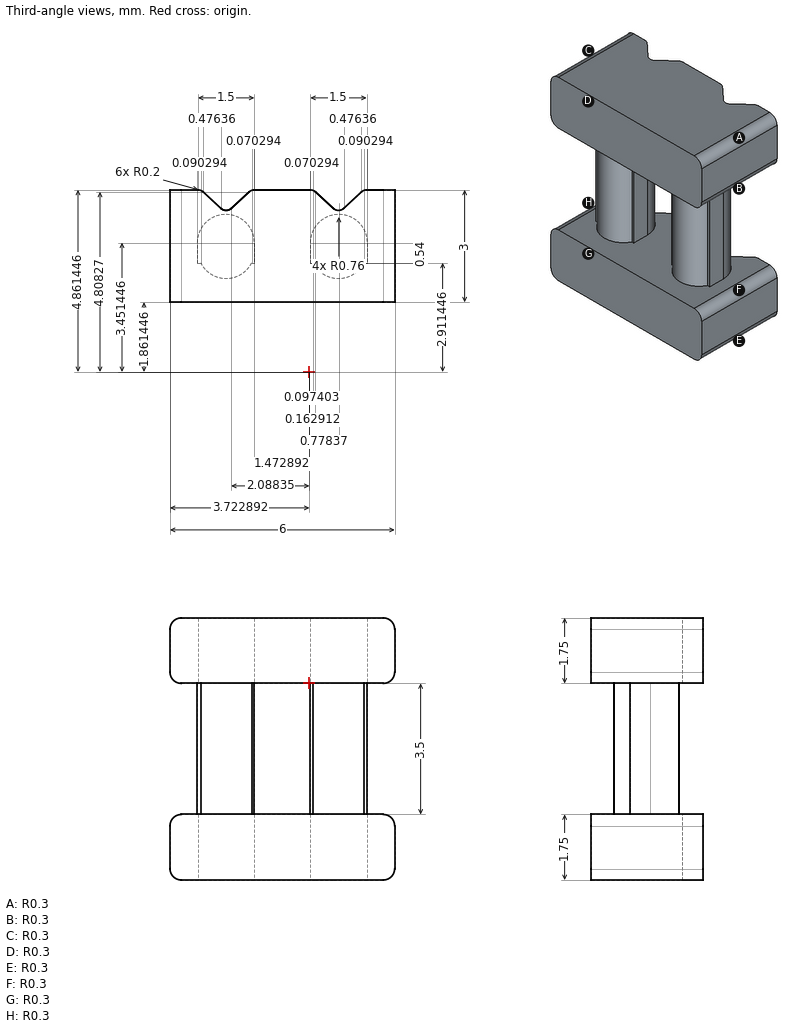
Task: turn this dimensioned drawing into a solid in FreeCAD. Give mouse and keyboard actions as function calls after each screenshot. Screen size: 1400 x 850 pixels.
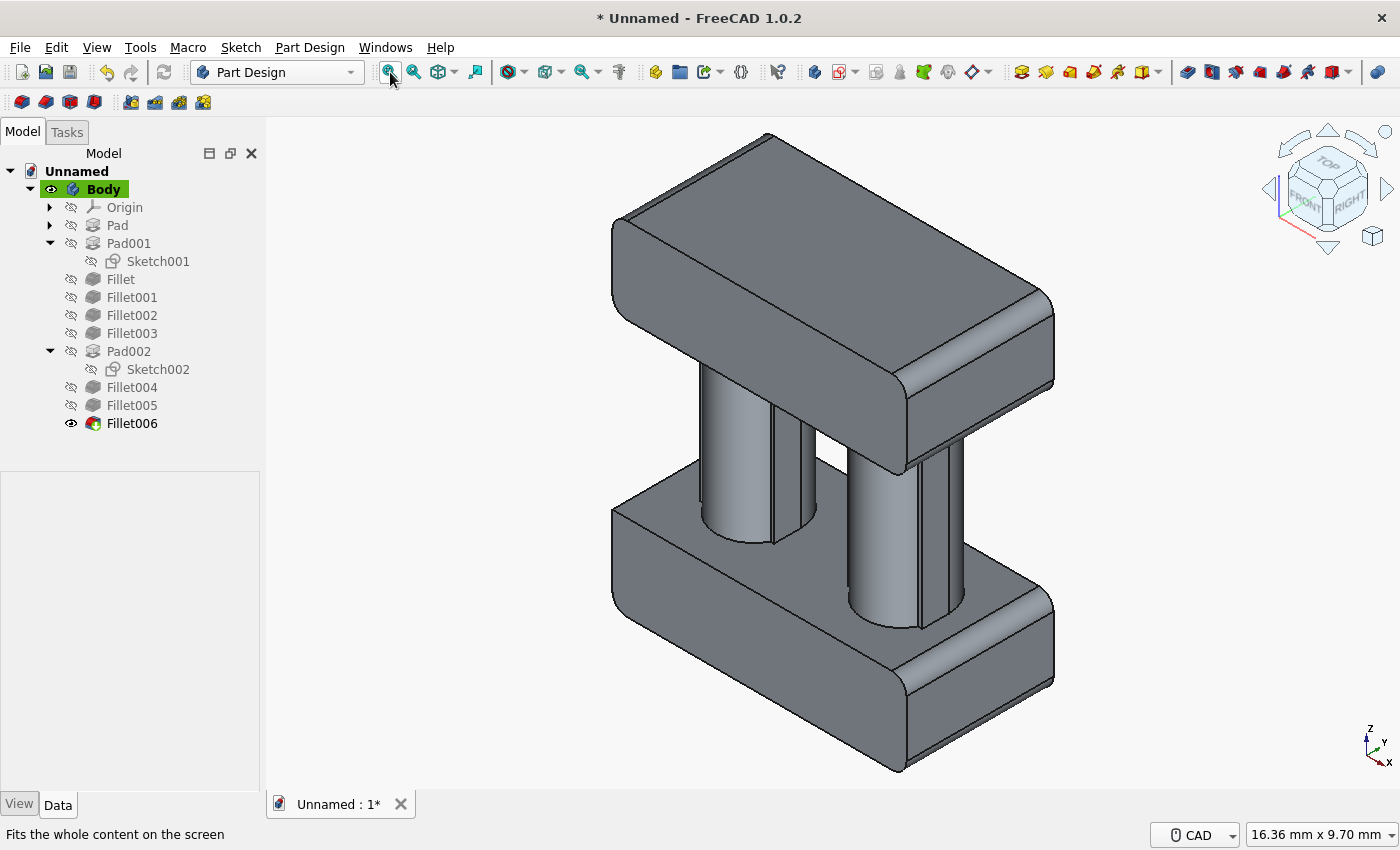
key(2)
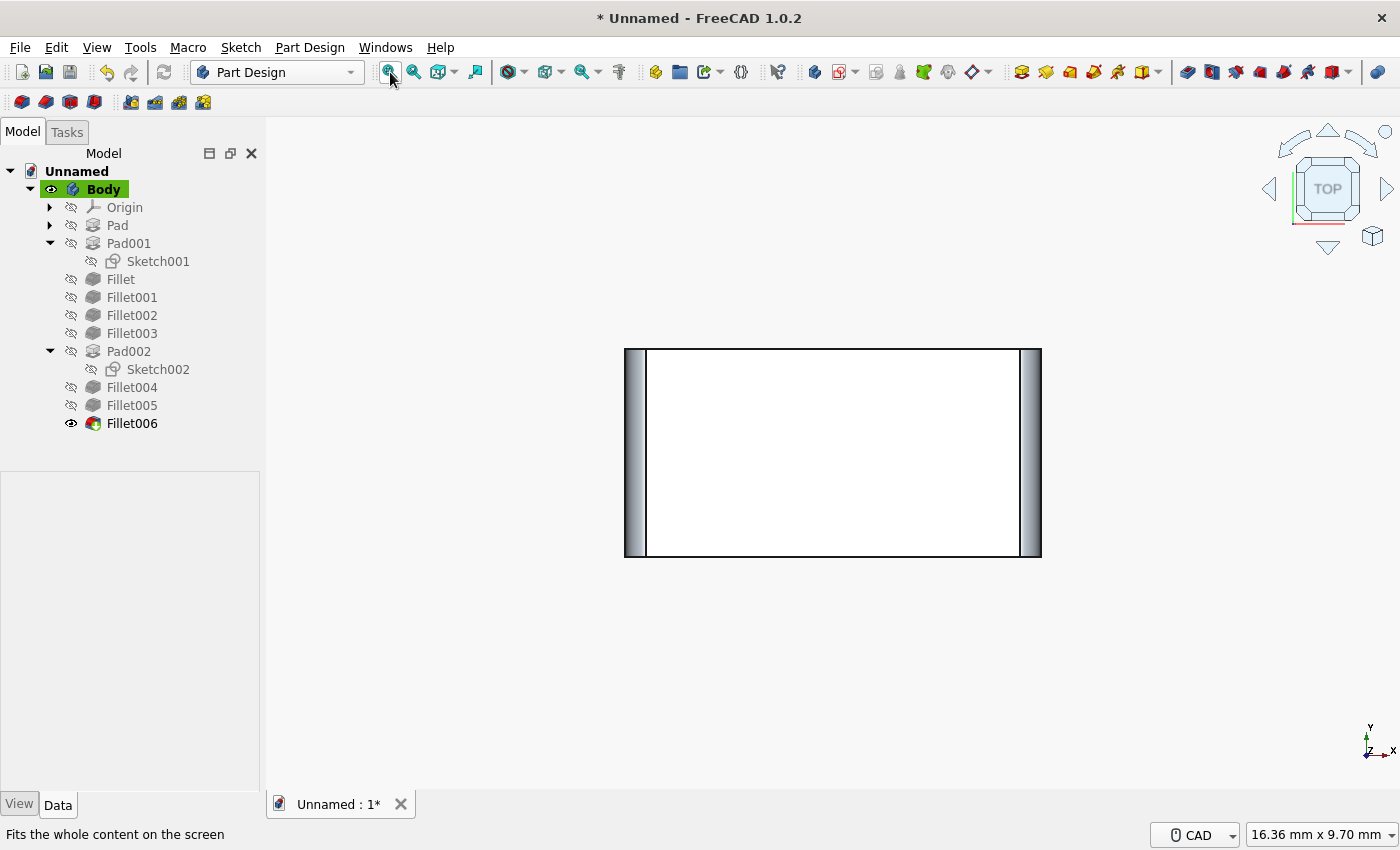
click(390, 72)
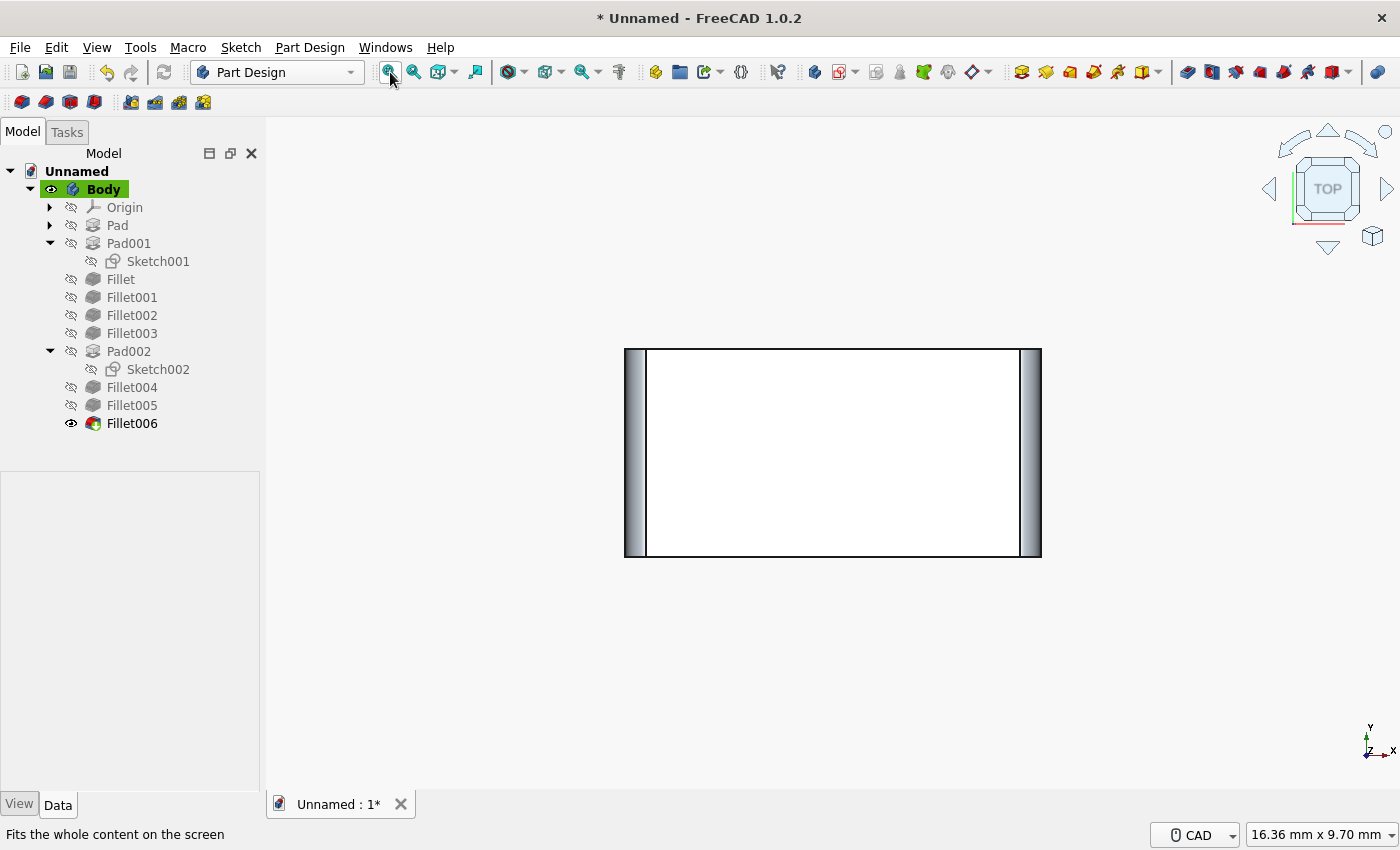
key(1)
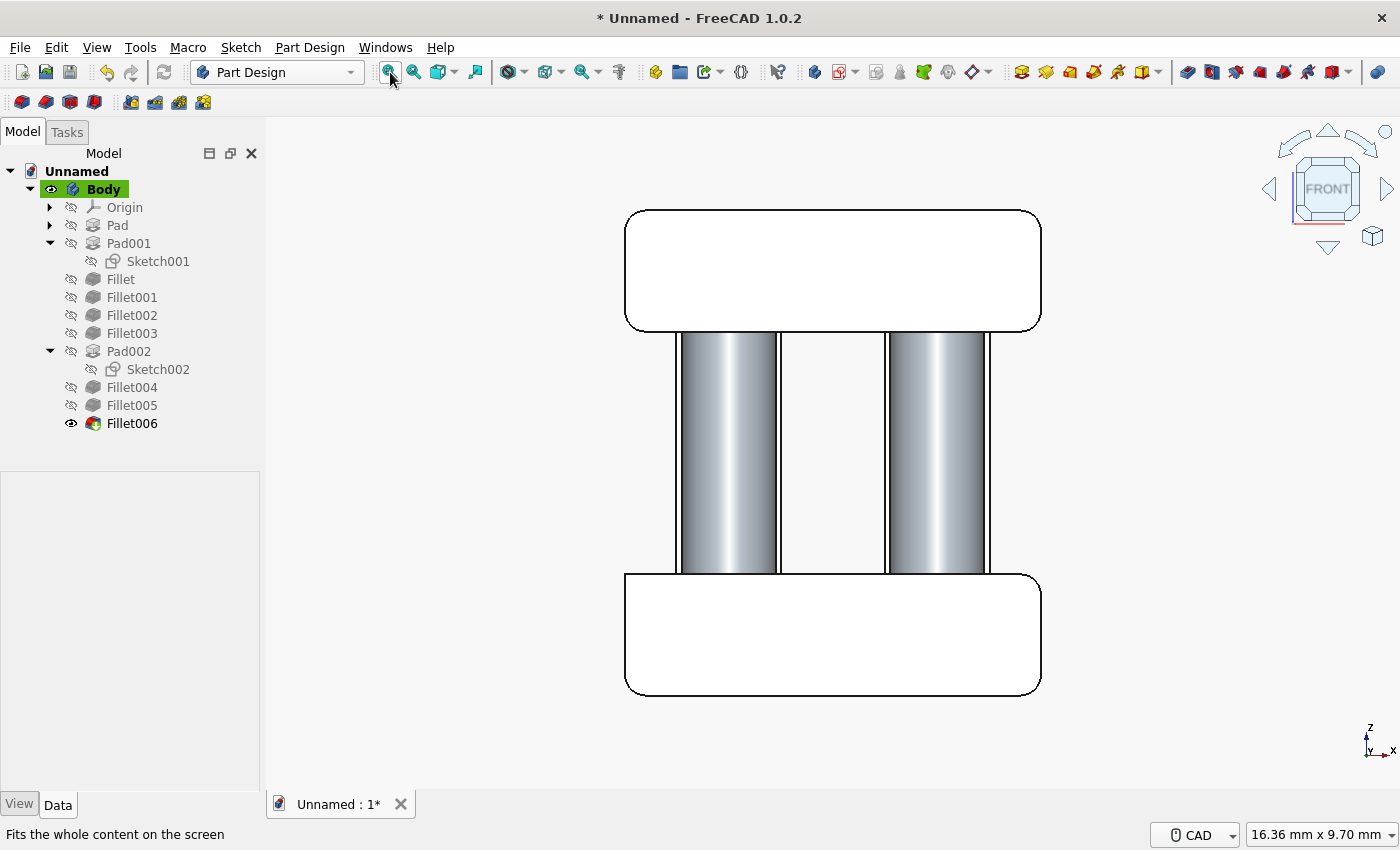
key(3)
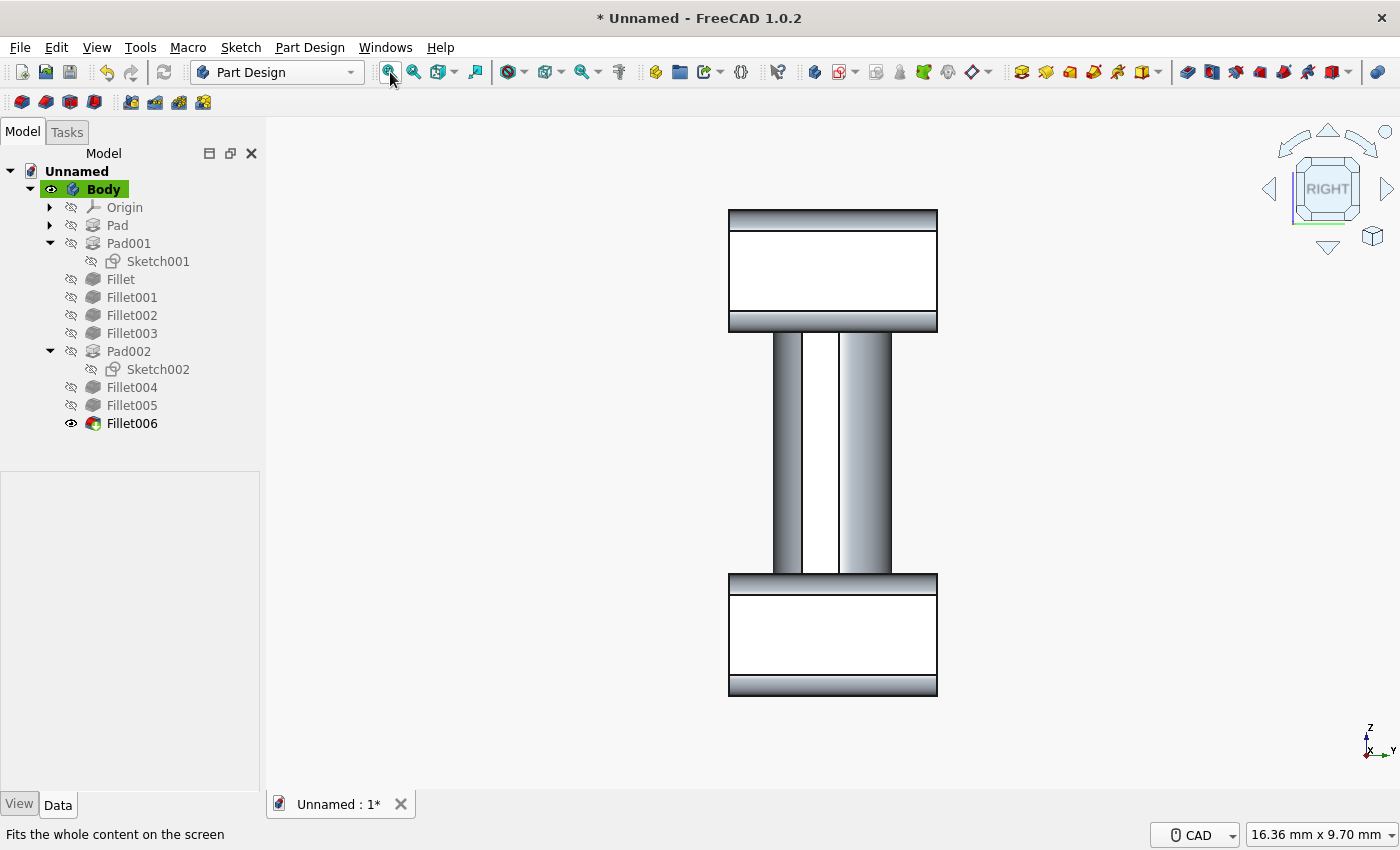
key(5)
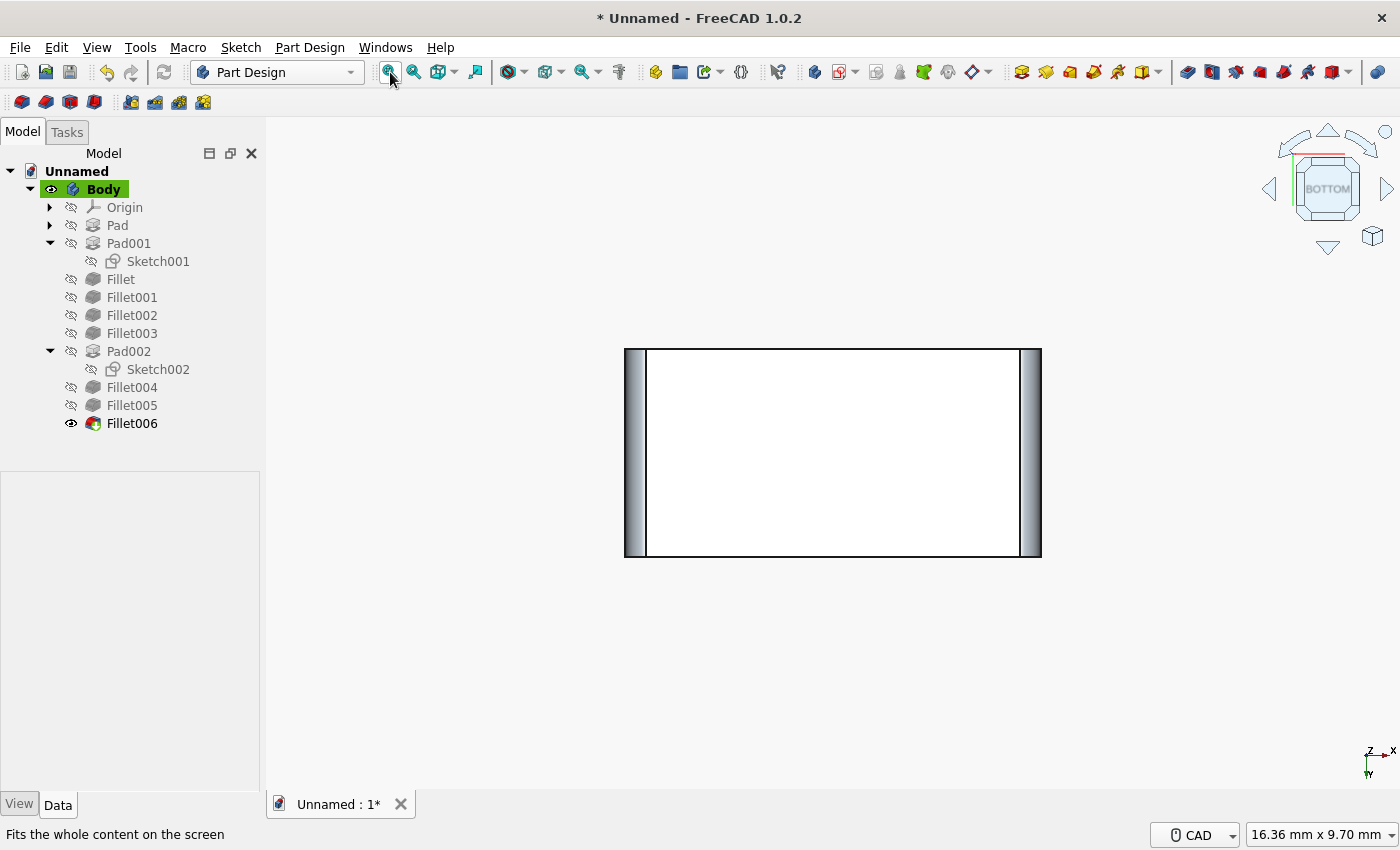
click(390, 72)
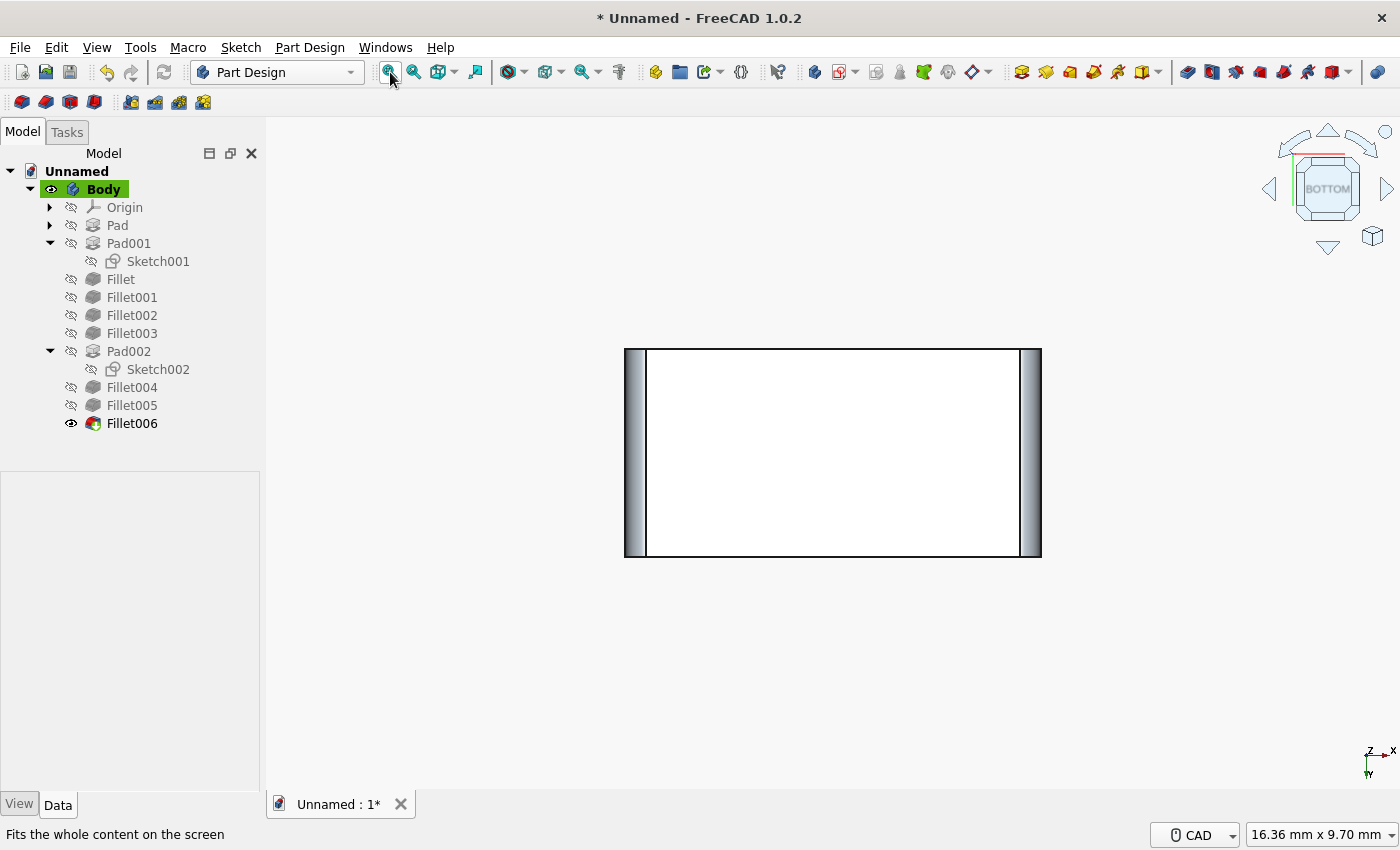
key(4)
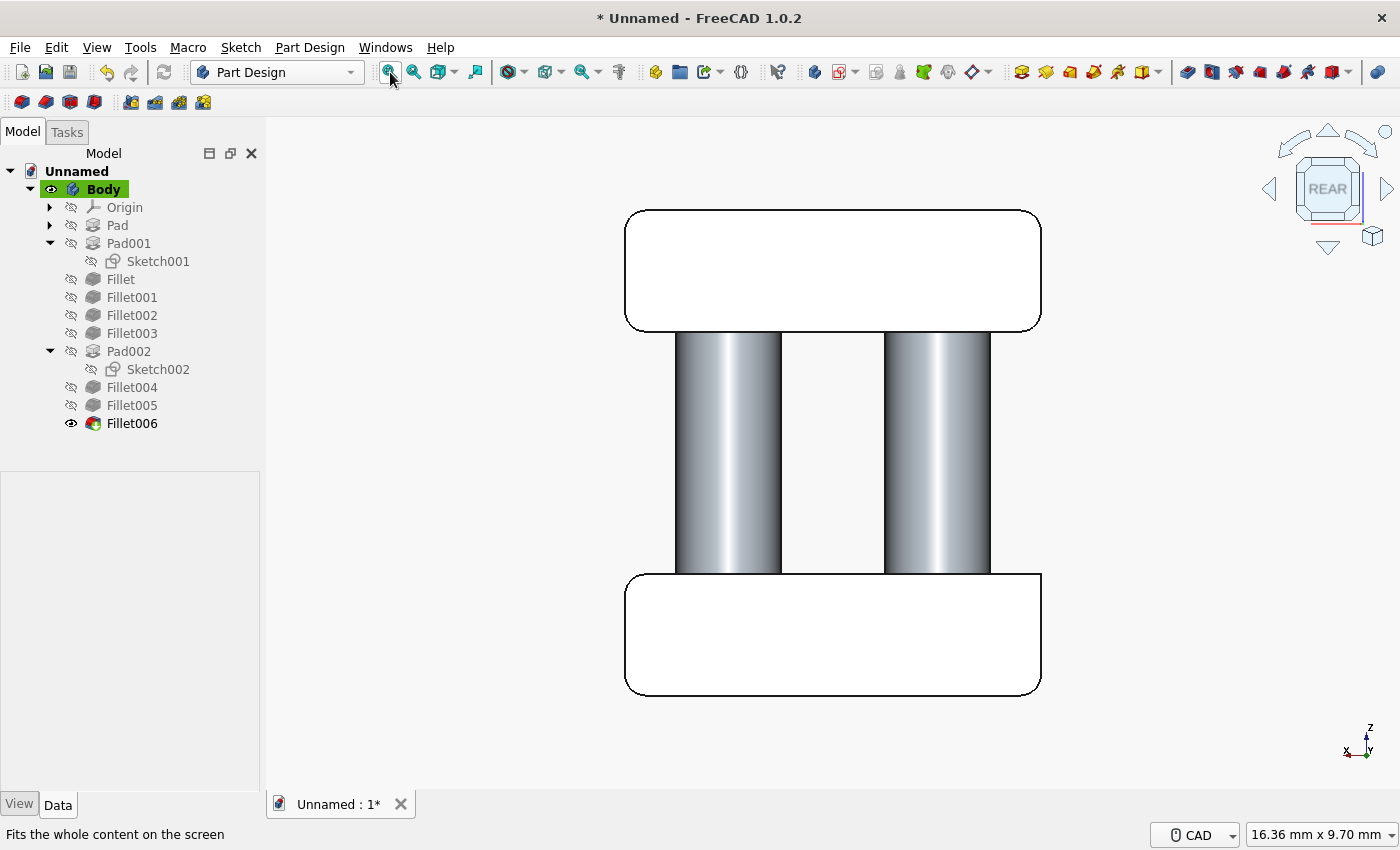
key(6)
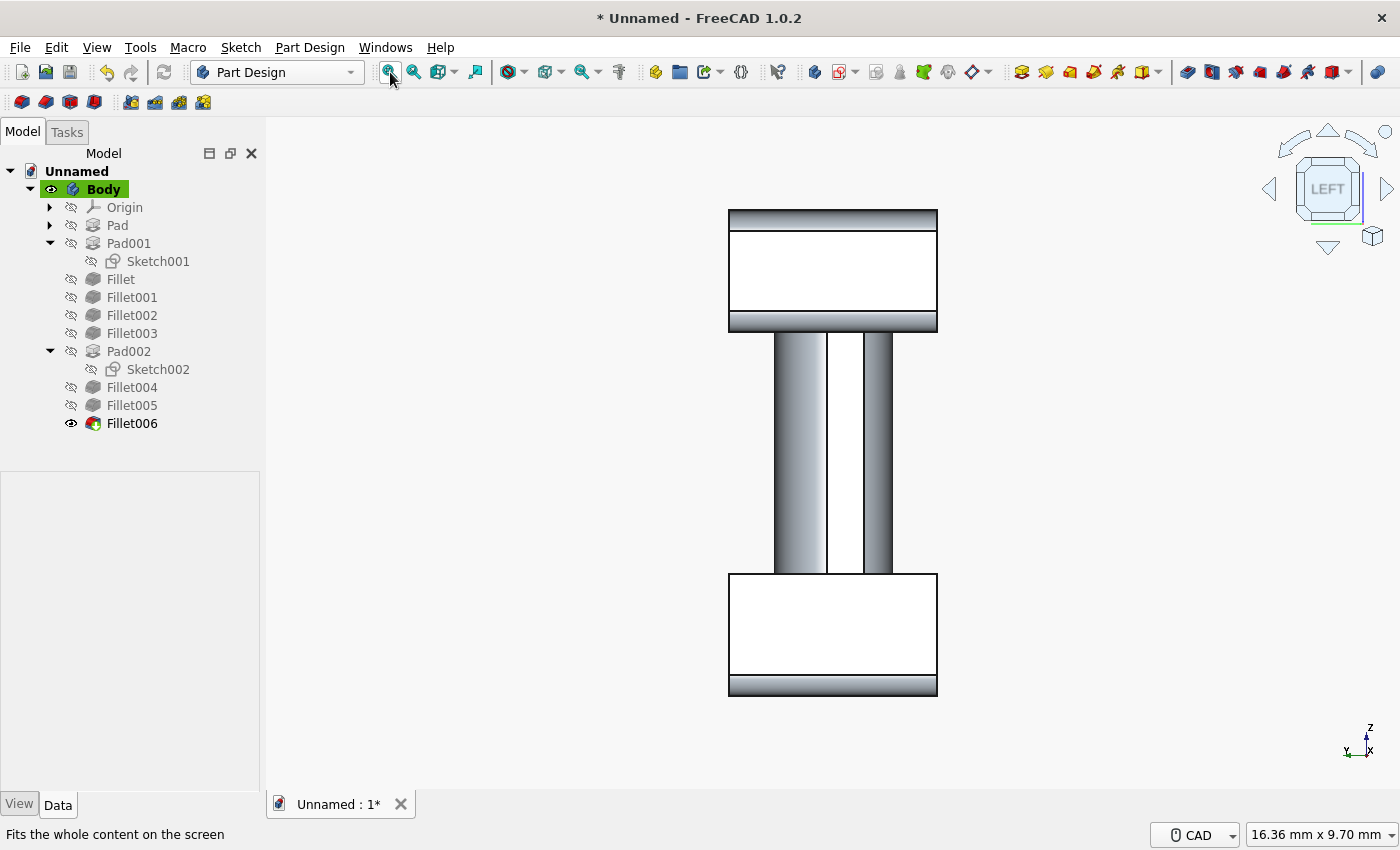
click(833, 573)